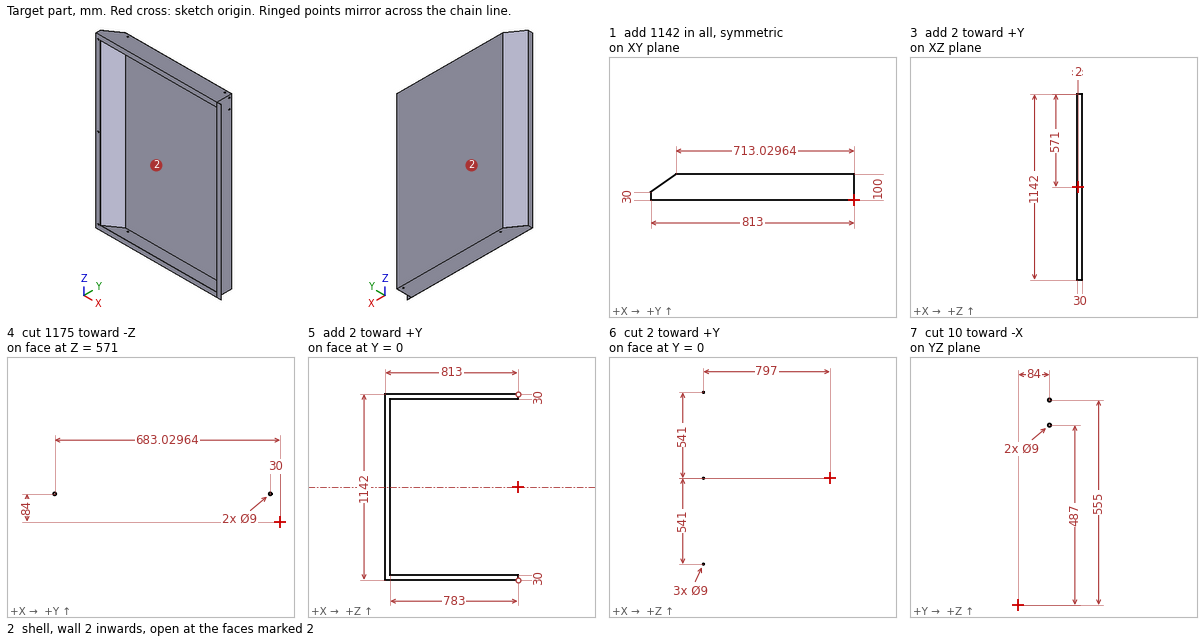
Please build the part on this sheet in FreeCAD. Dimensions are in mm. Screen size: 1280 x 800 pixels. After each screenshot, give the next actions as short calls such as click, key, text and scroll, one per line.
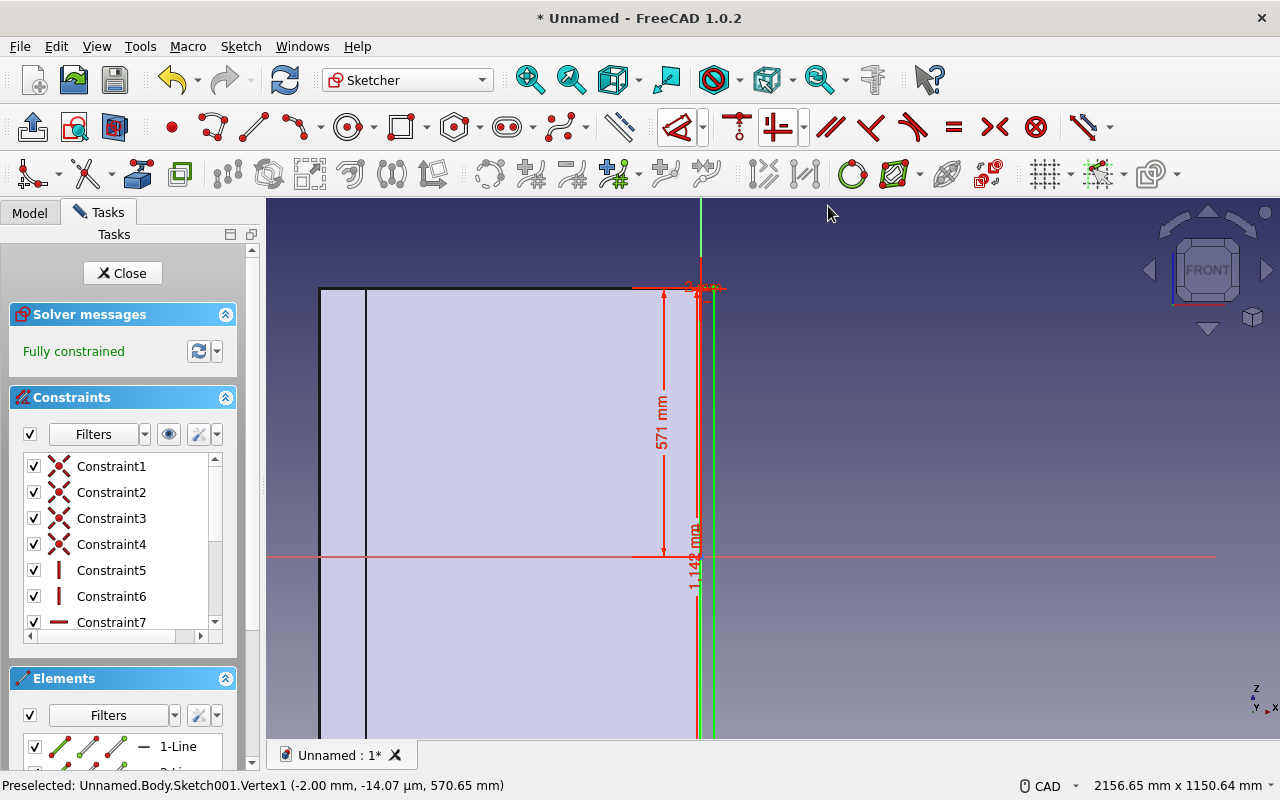
click(123, 273)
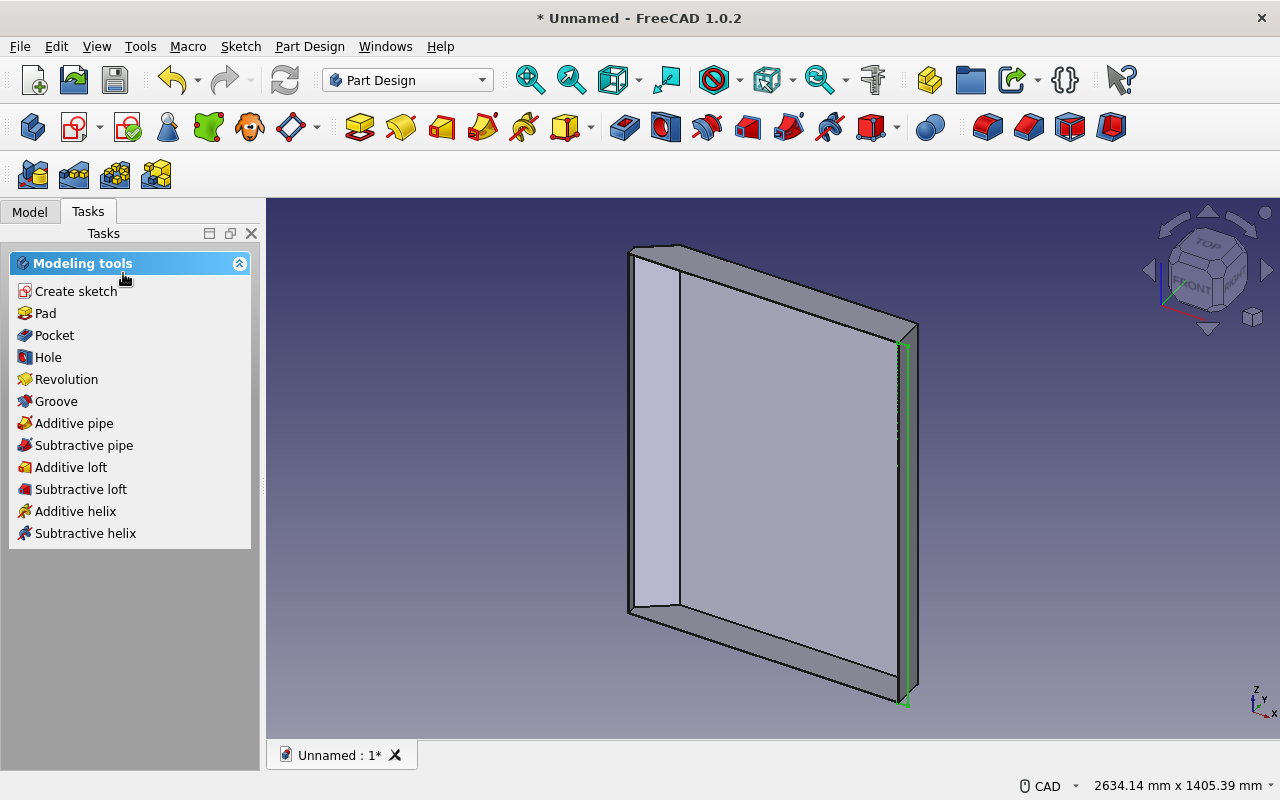
click(360, 128)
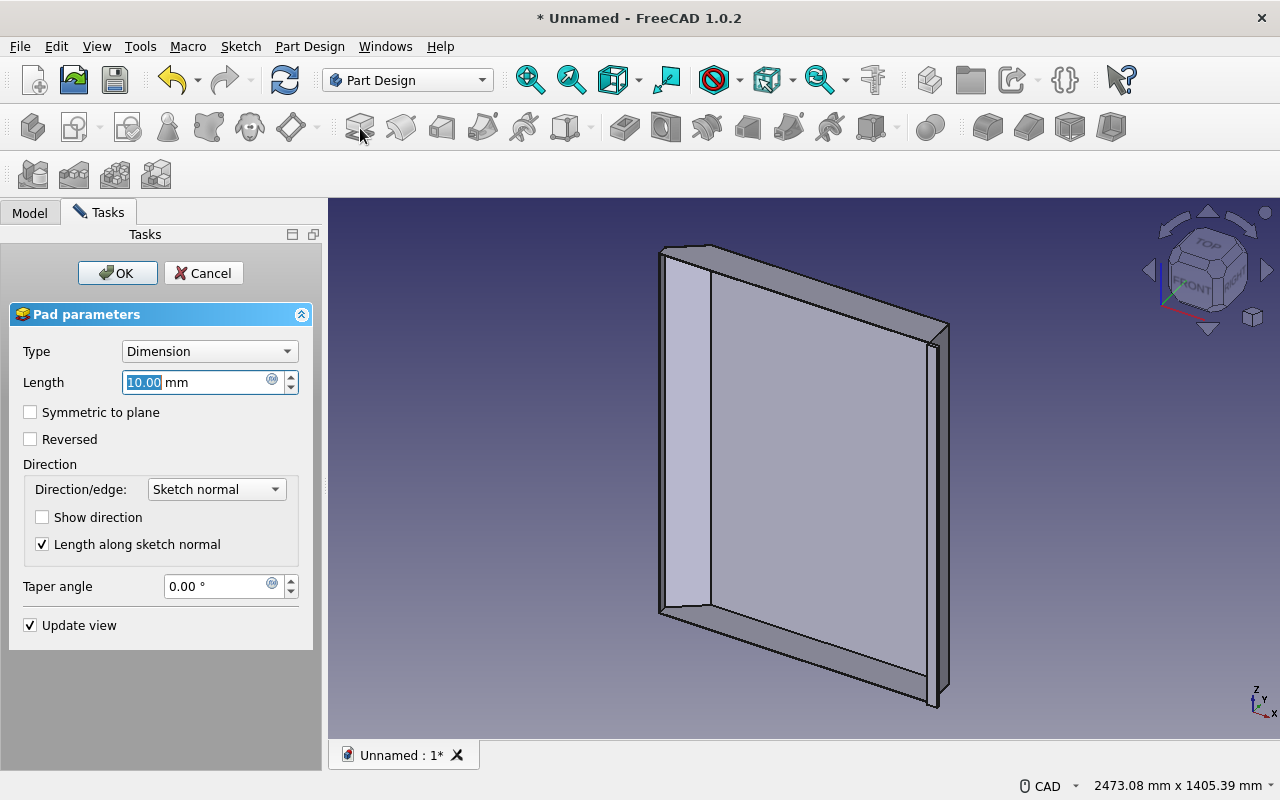
text(2)
key(Tab)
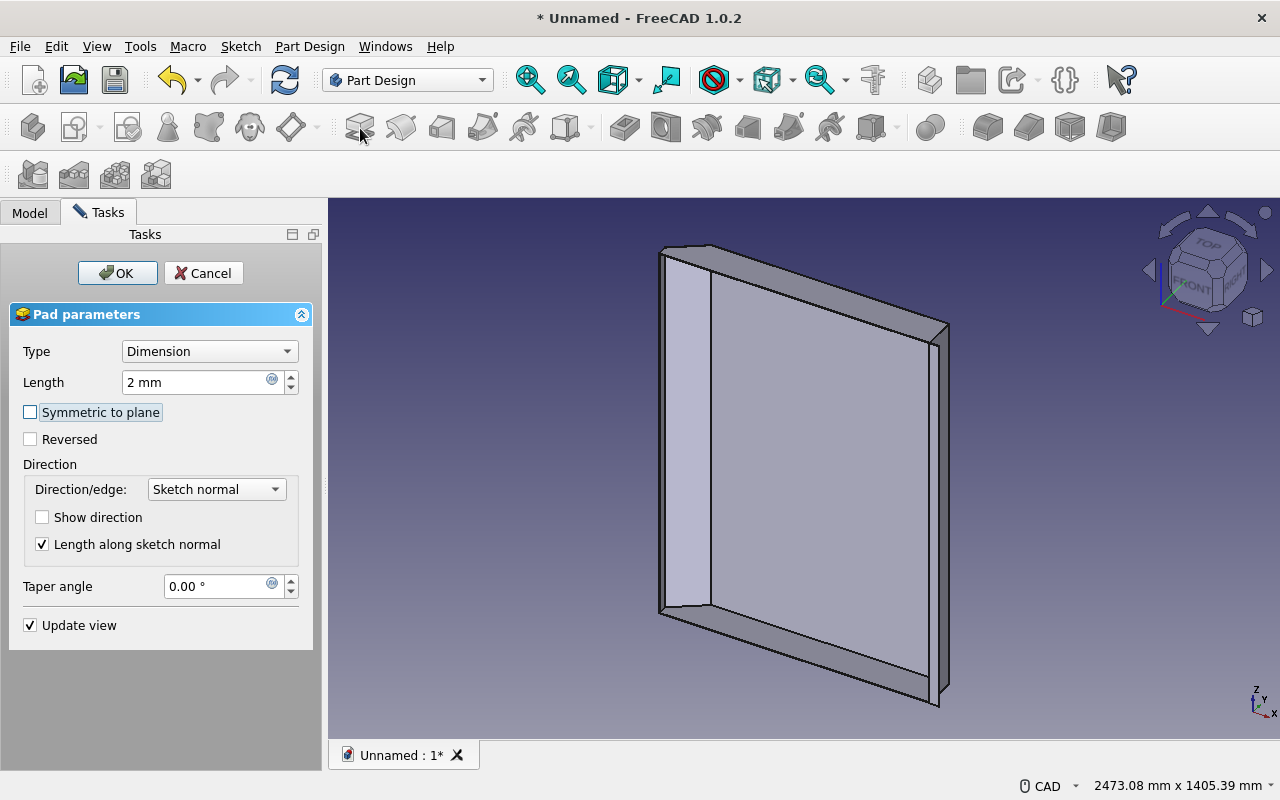
click(31, 439)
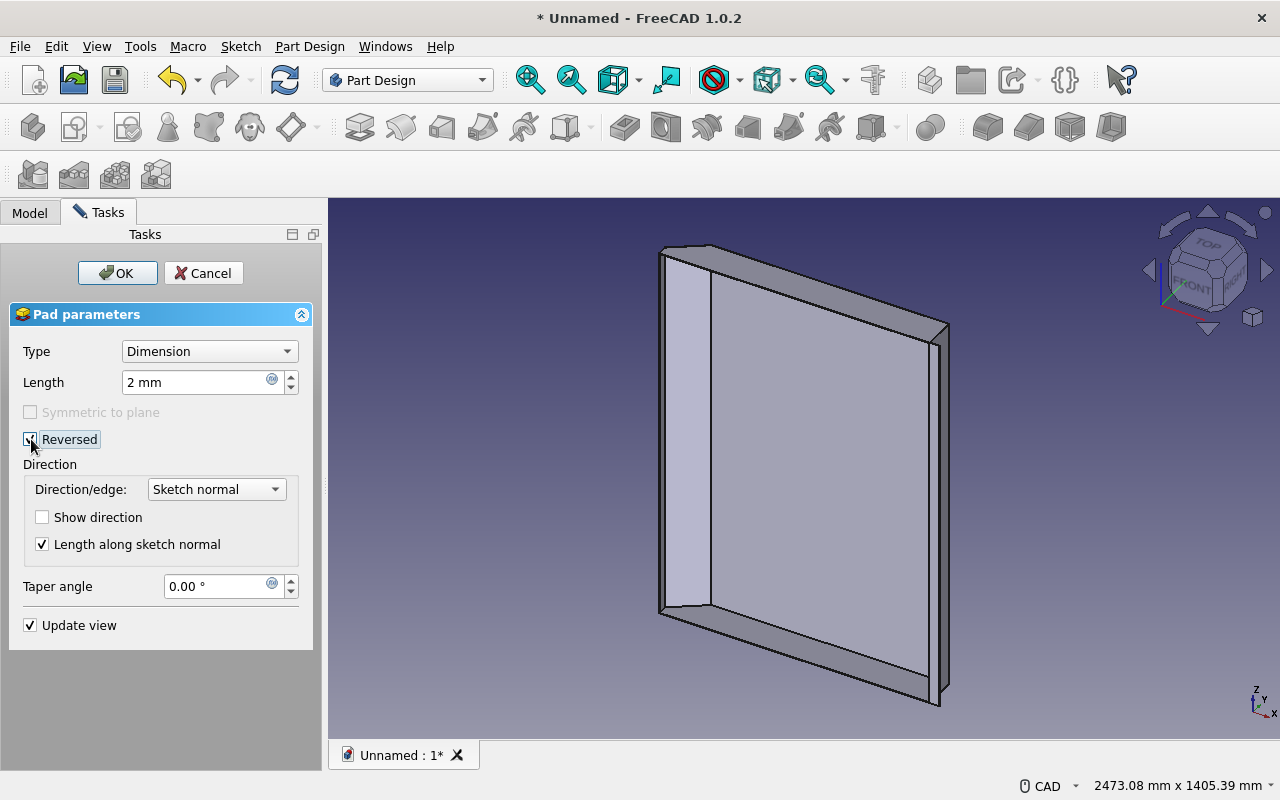
click(118, 273)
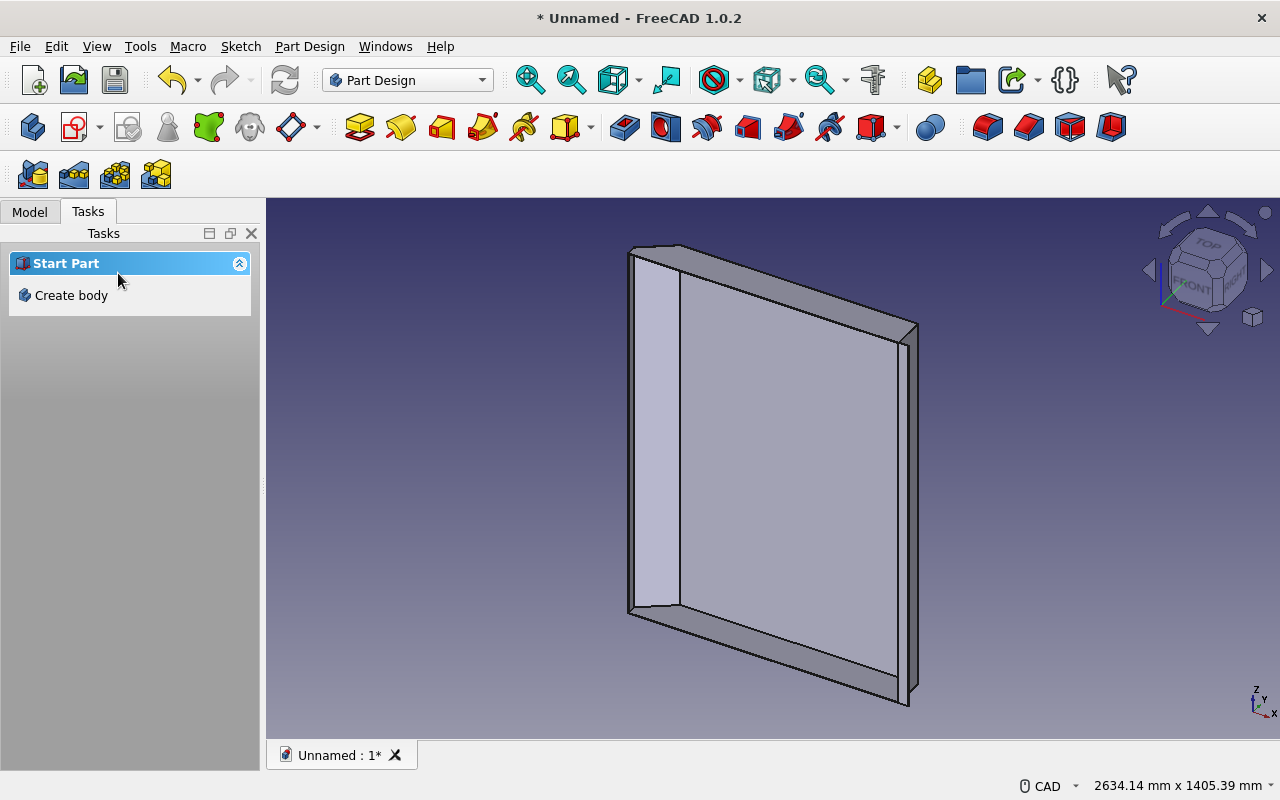
click(858, 316)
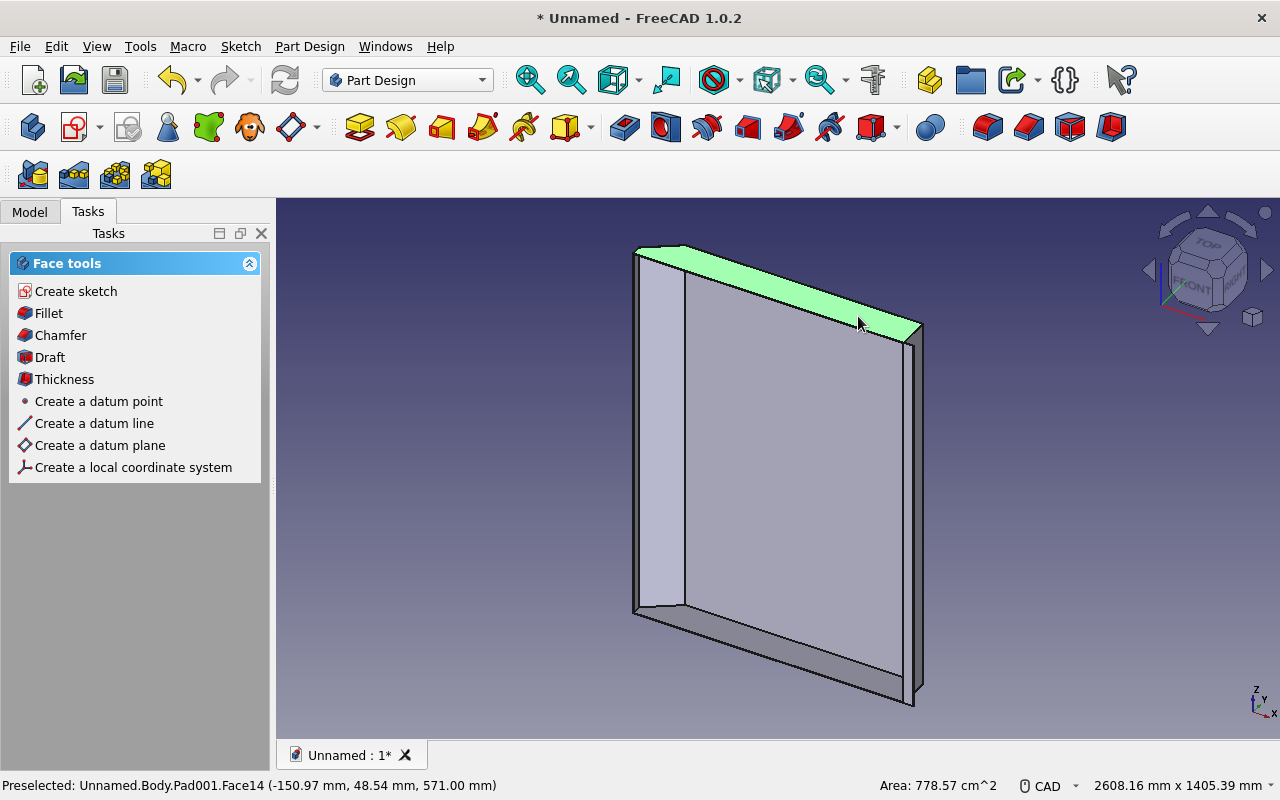
click(74, 128)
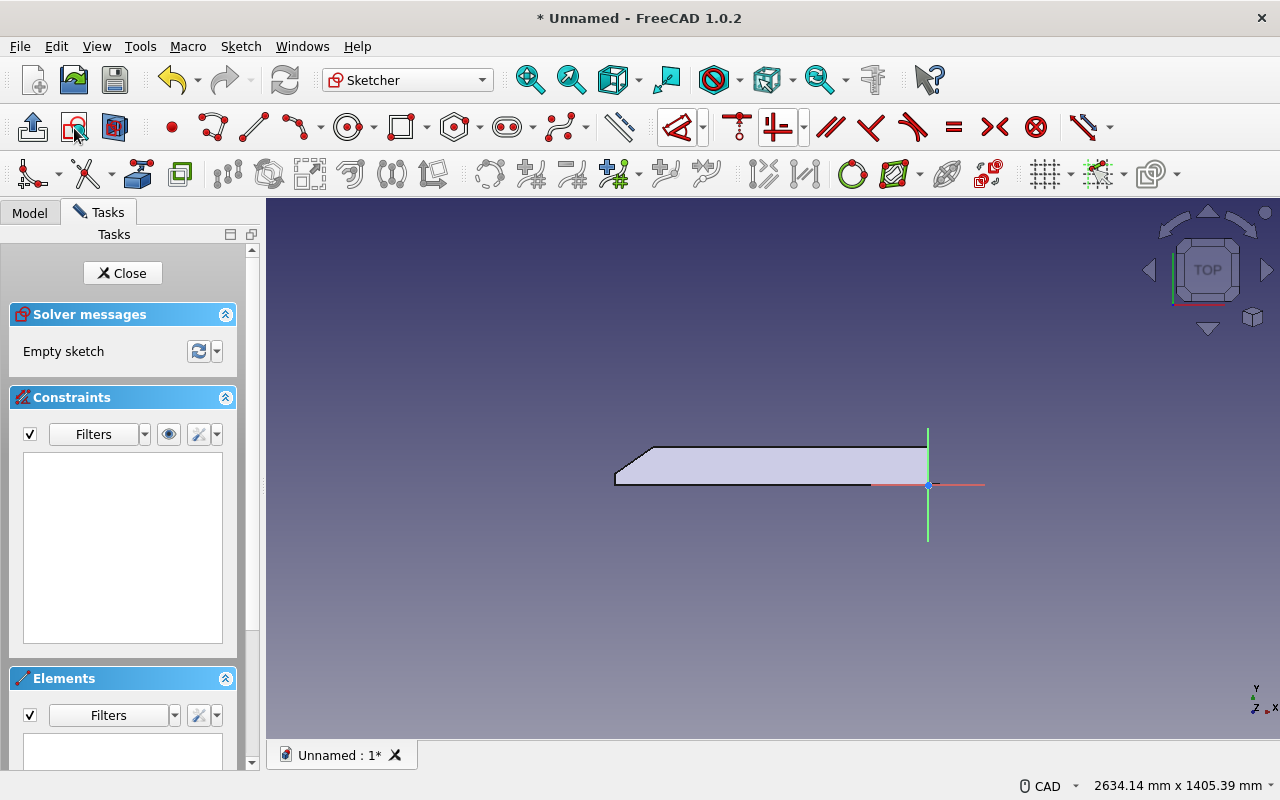
scroll(870, 468, up, 4)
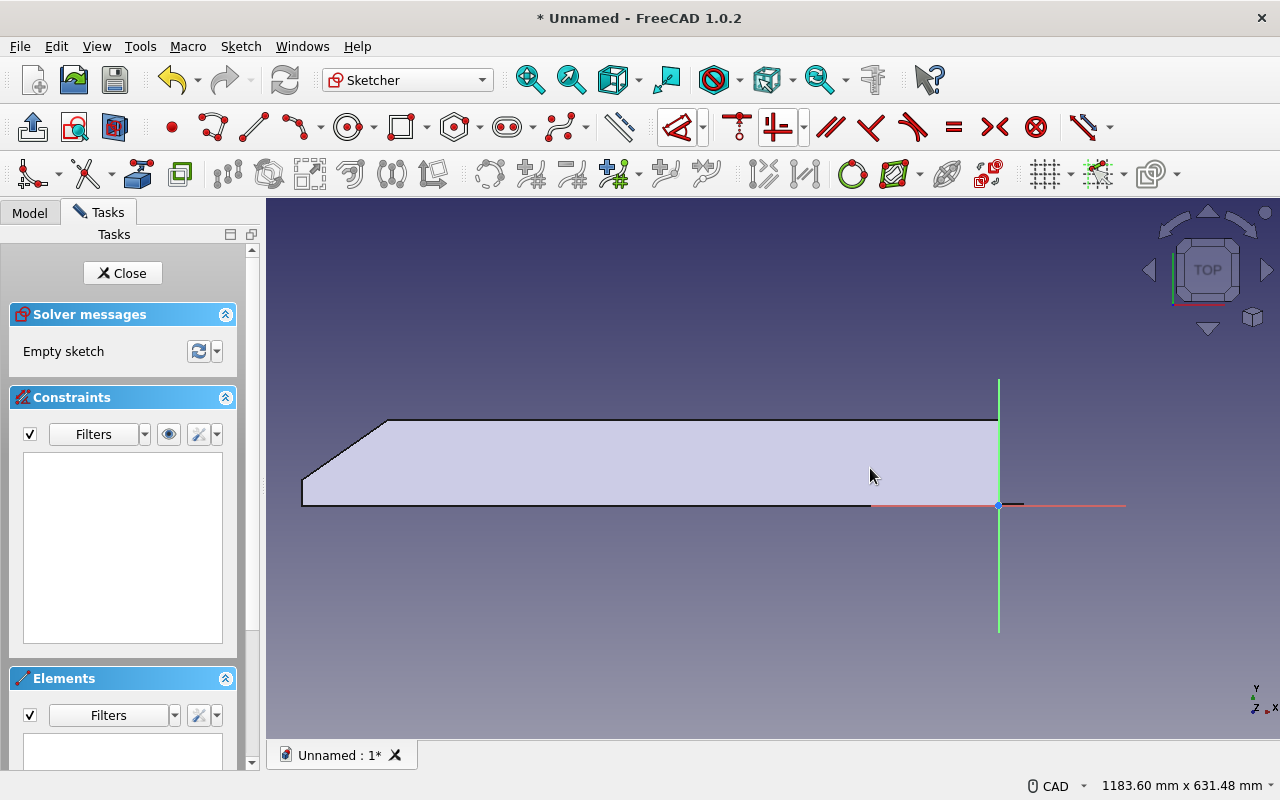
key(g)
key(c)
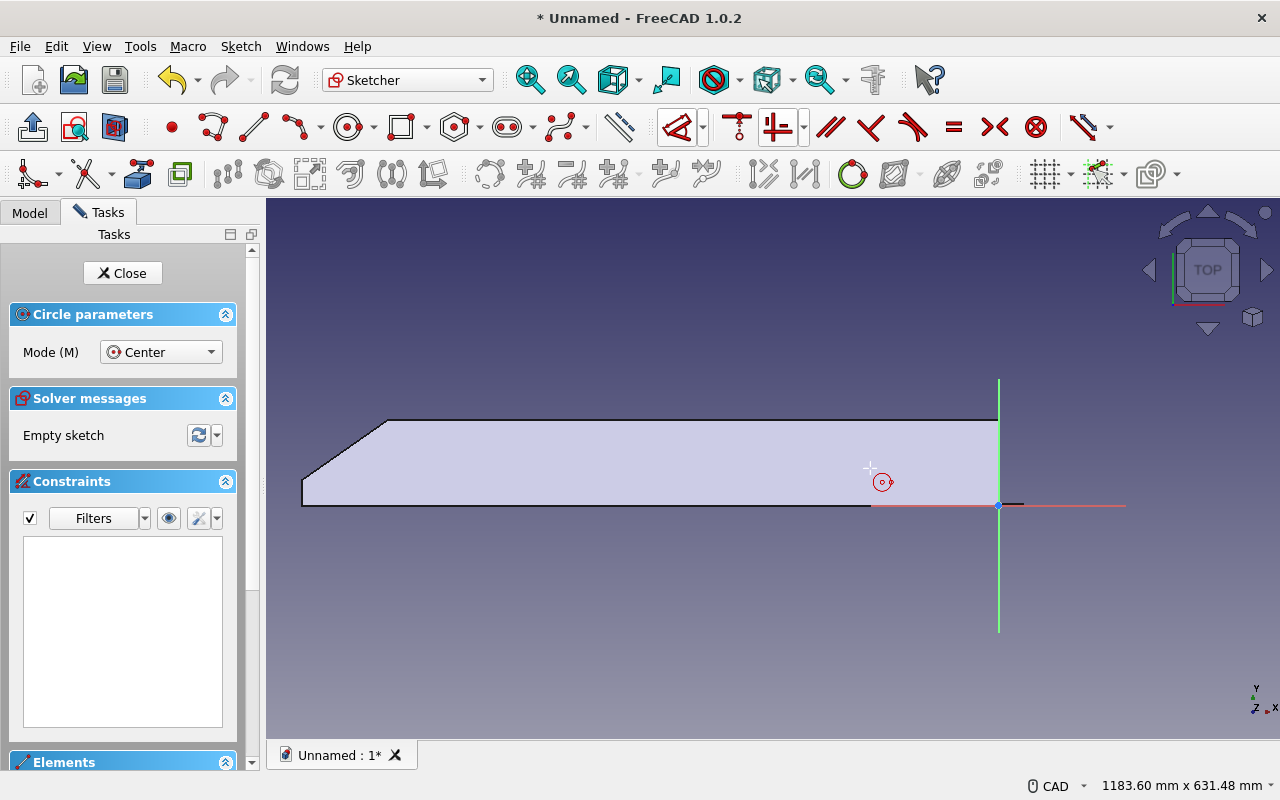
scroll(413, 434, up, 9)